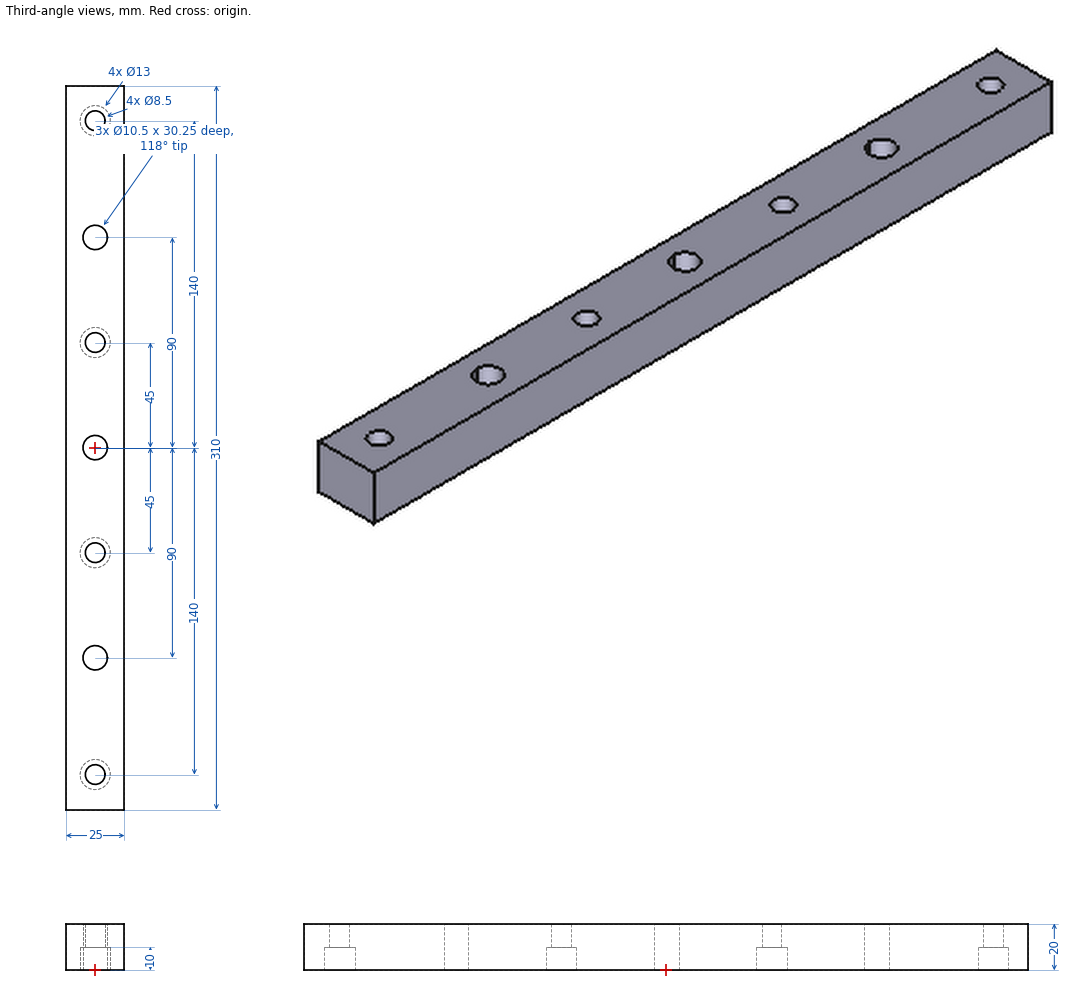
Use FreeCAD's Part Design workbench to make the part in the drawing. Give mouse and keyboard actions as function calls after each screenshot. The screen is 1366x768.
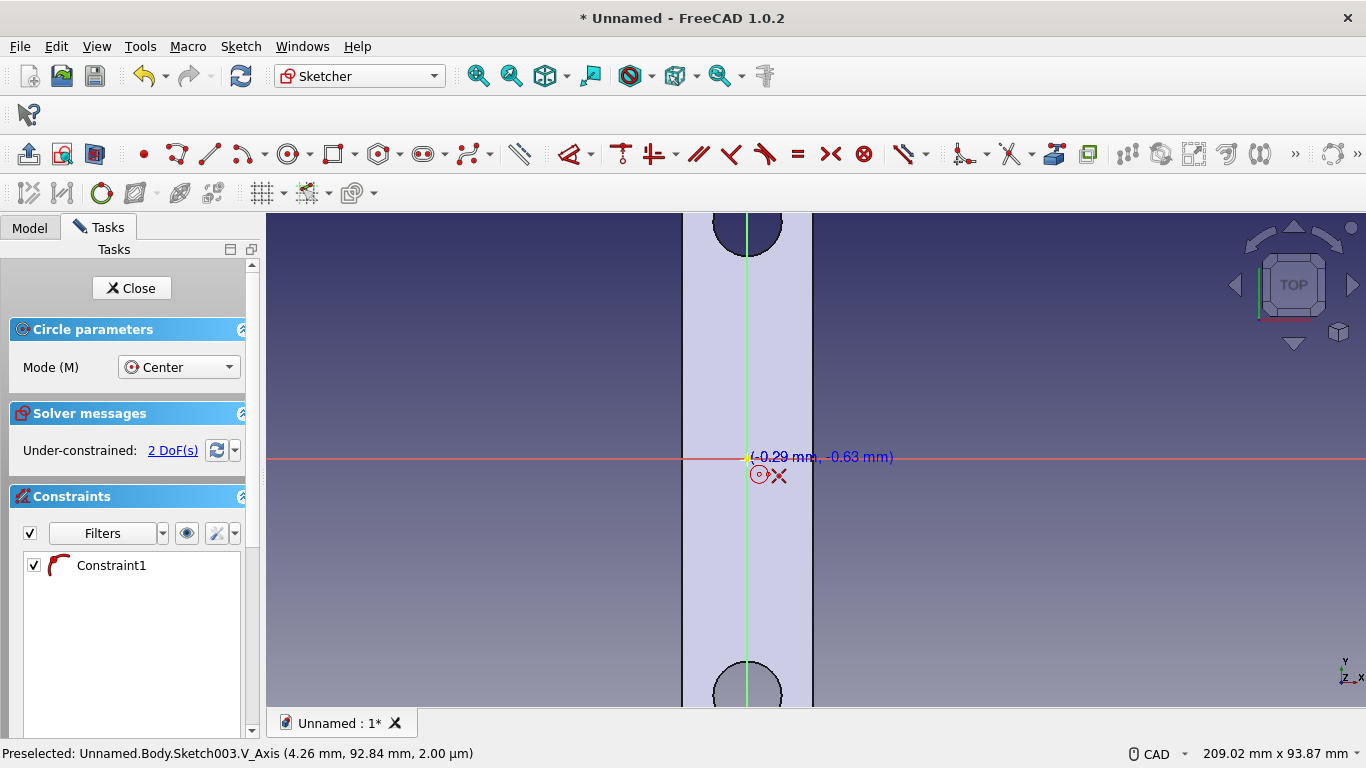
click(747, 459)
click(767, 439)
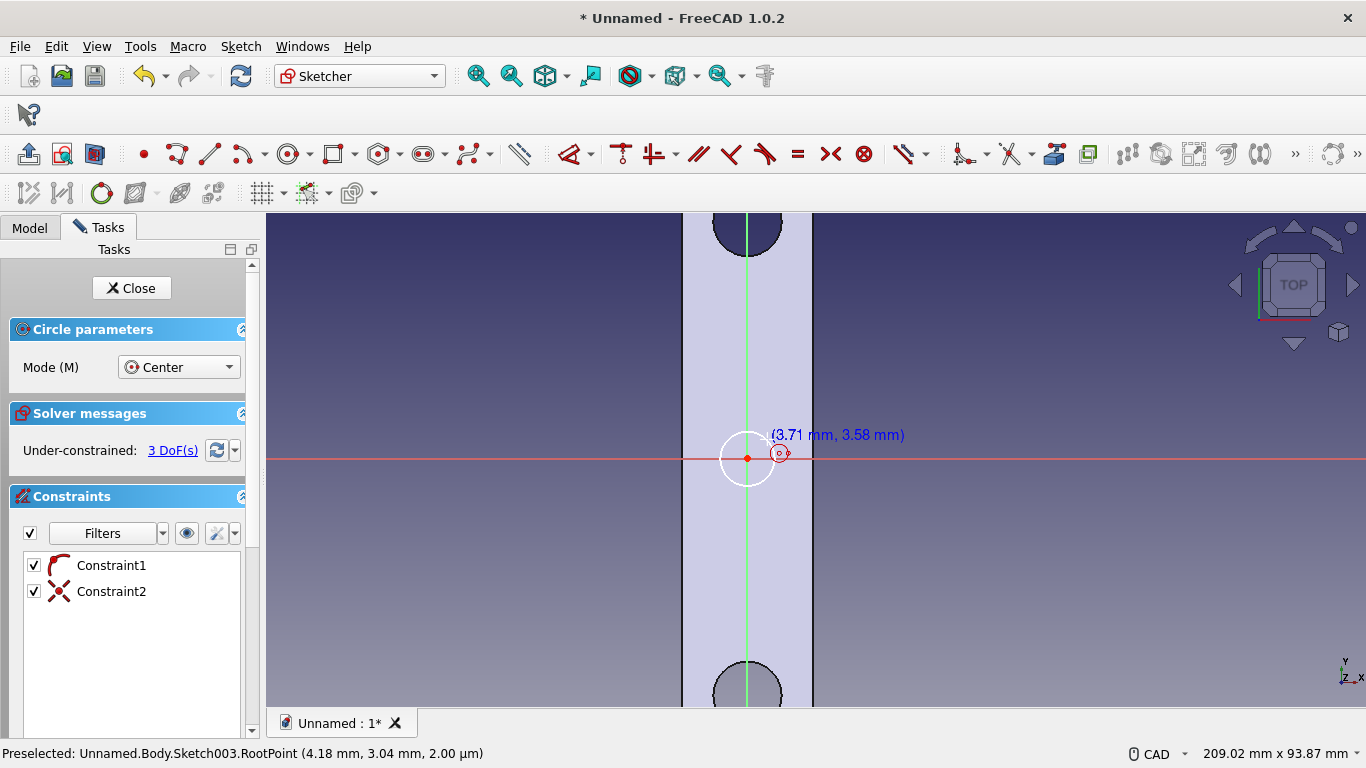
scroll(748, 461, down, 6)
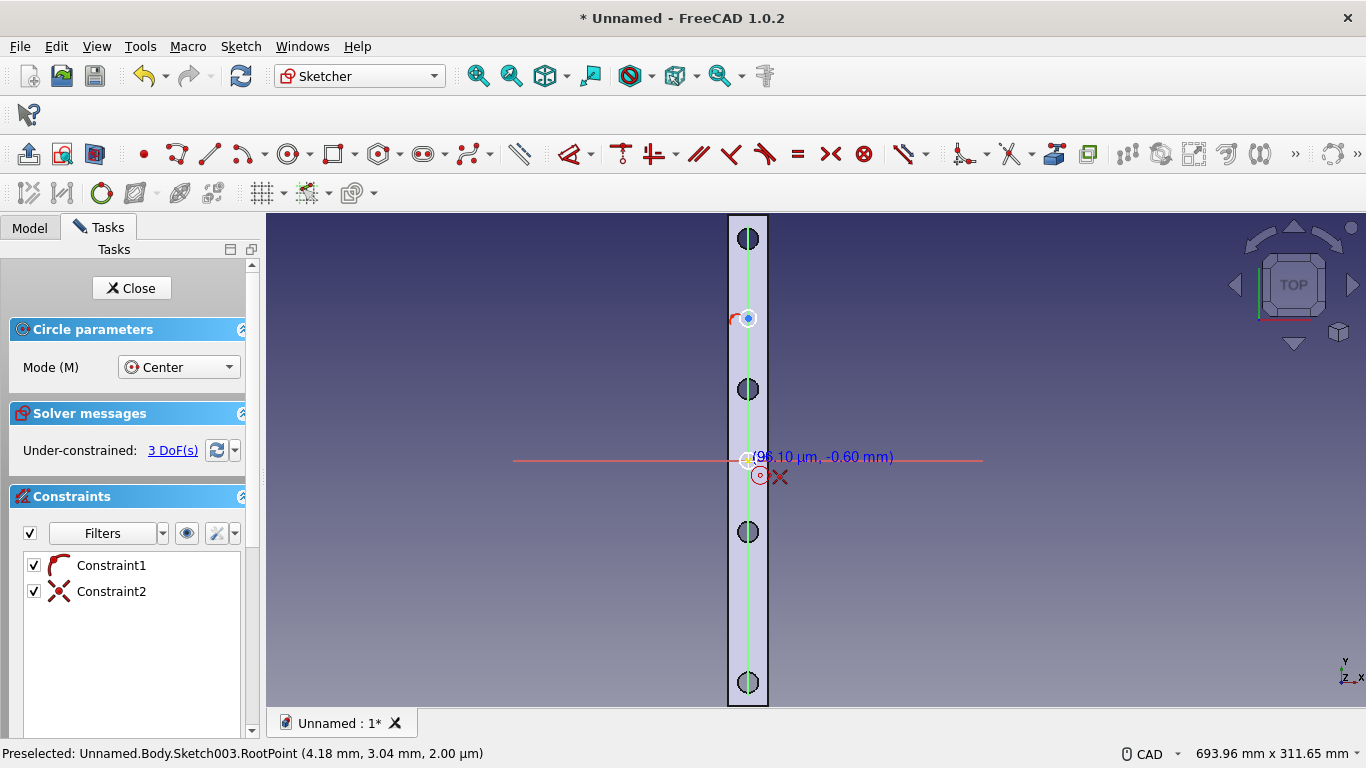
scroll(748, 603, up, 6)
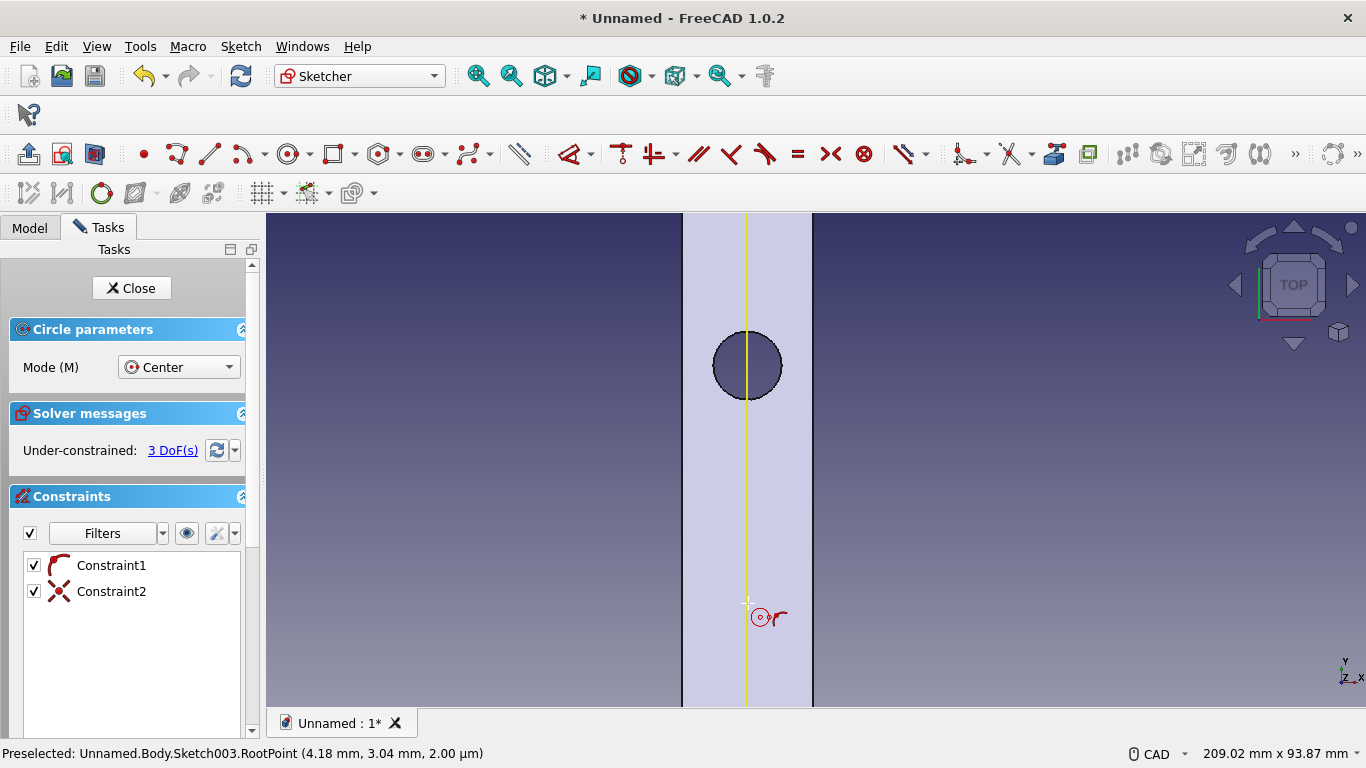
click(747, 602)
click(767, 583)
key(Escape)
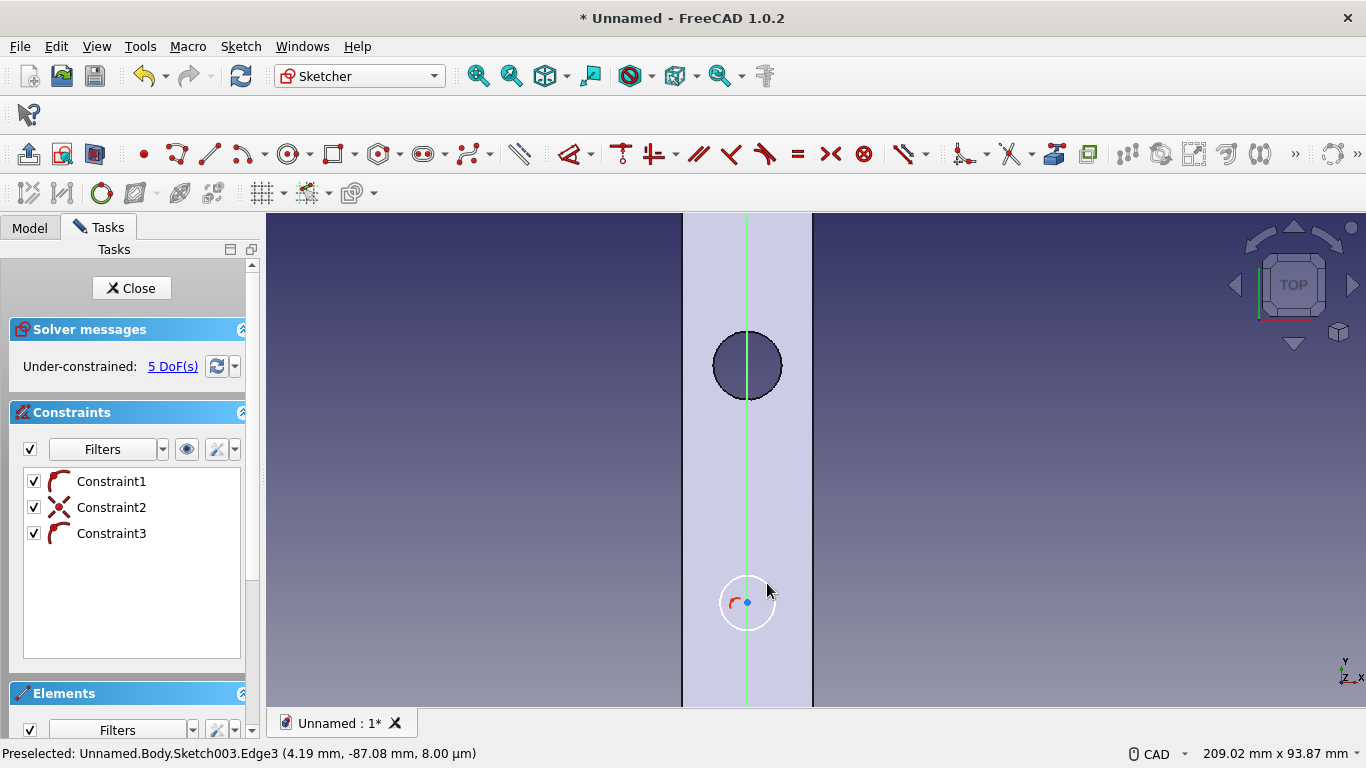
scroll(748, 603, down, 6)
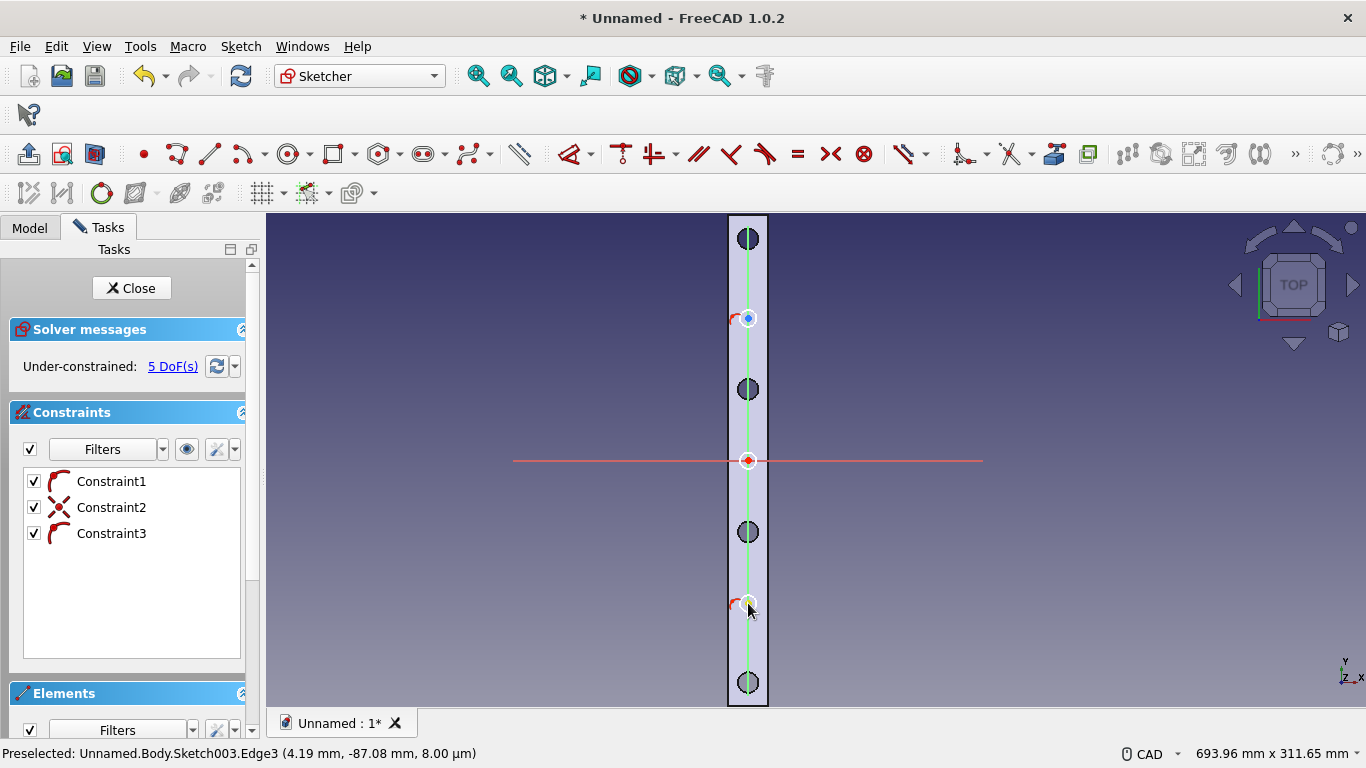
scroll(754, 313, up, 5)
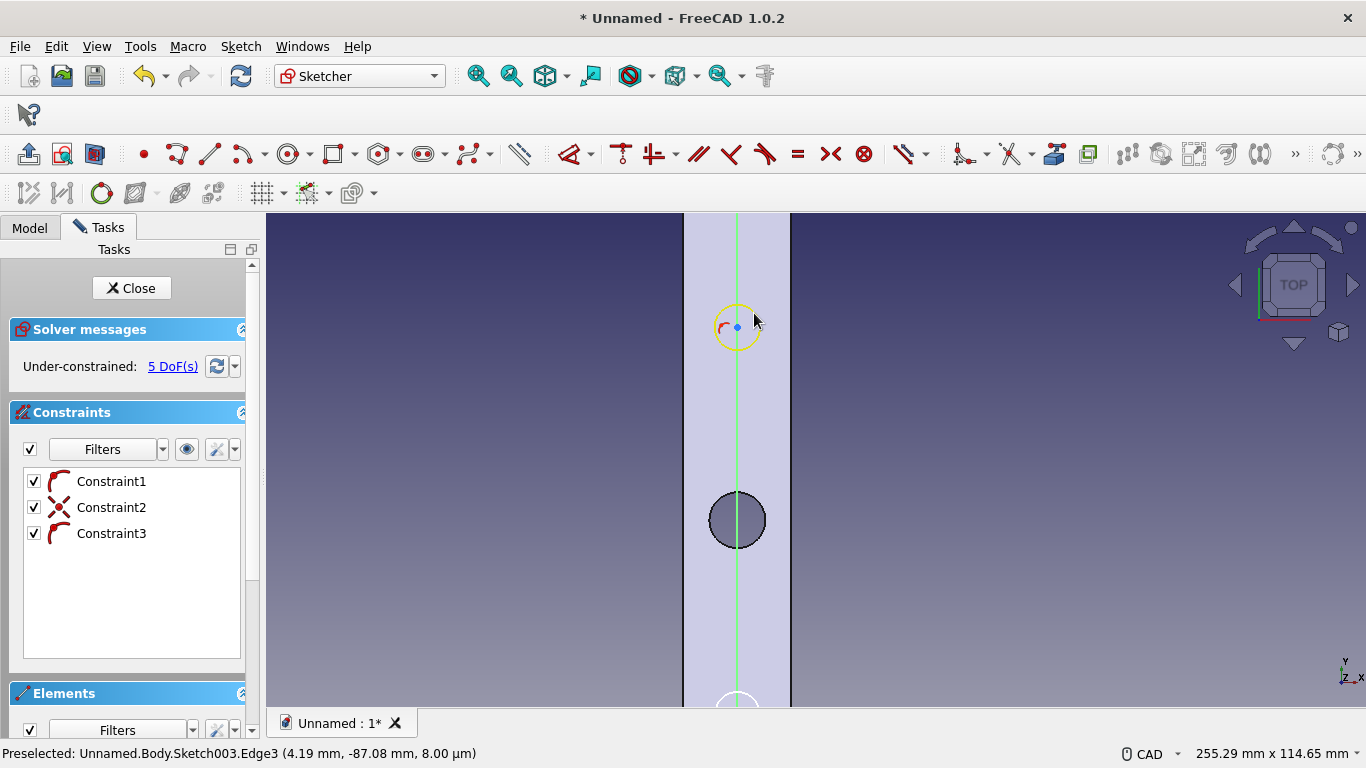
click(753, 311)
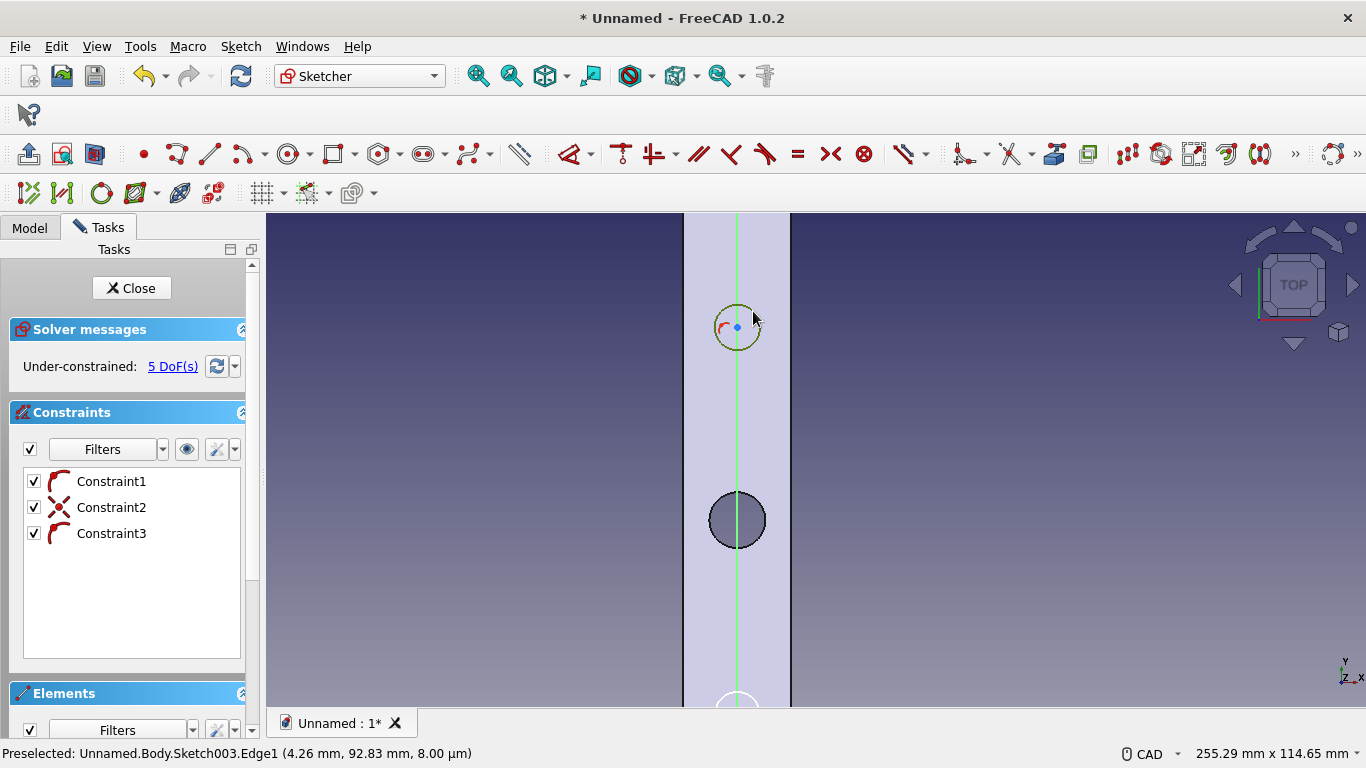
scroll(753, 312, down, 5)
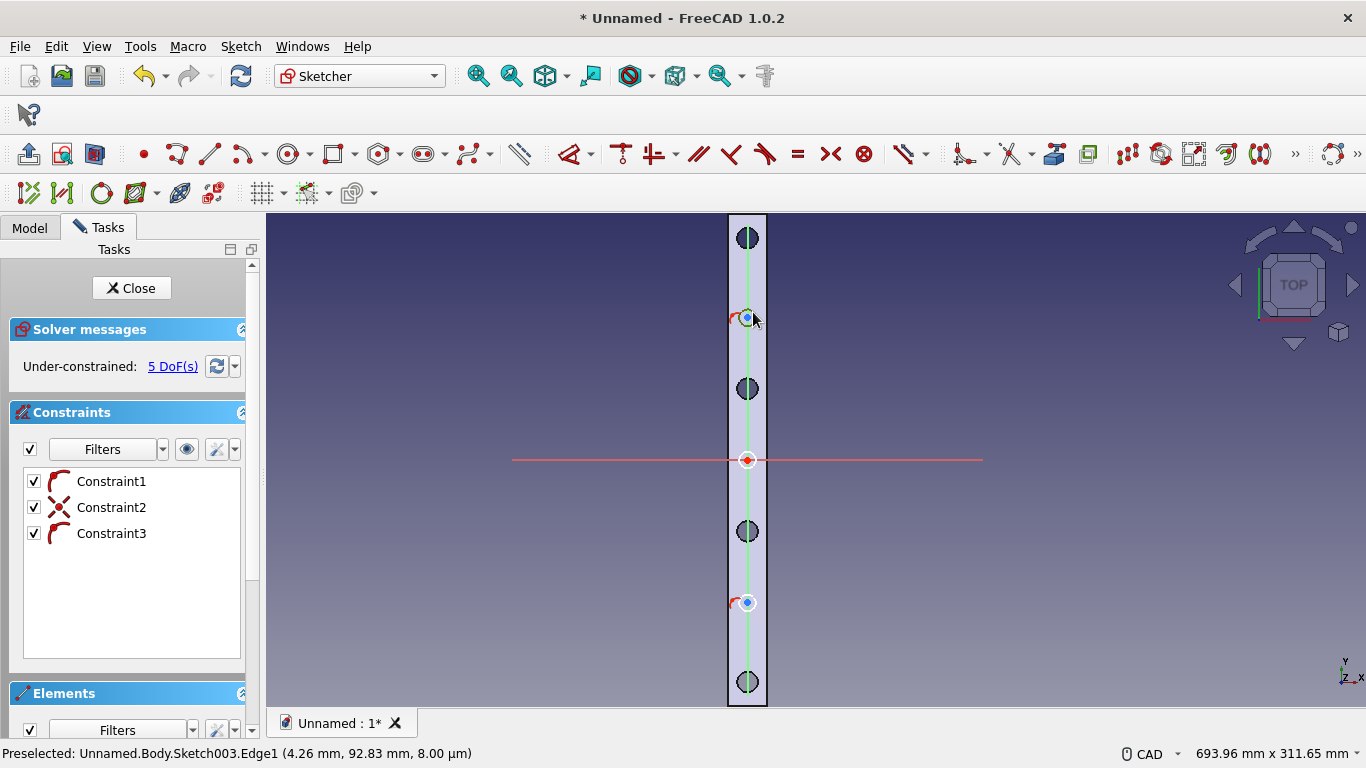
scroll(753, 454, up, 5)